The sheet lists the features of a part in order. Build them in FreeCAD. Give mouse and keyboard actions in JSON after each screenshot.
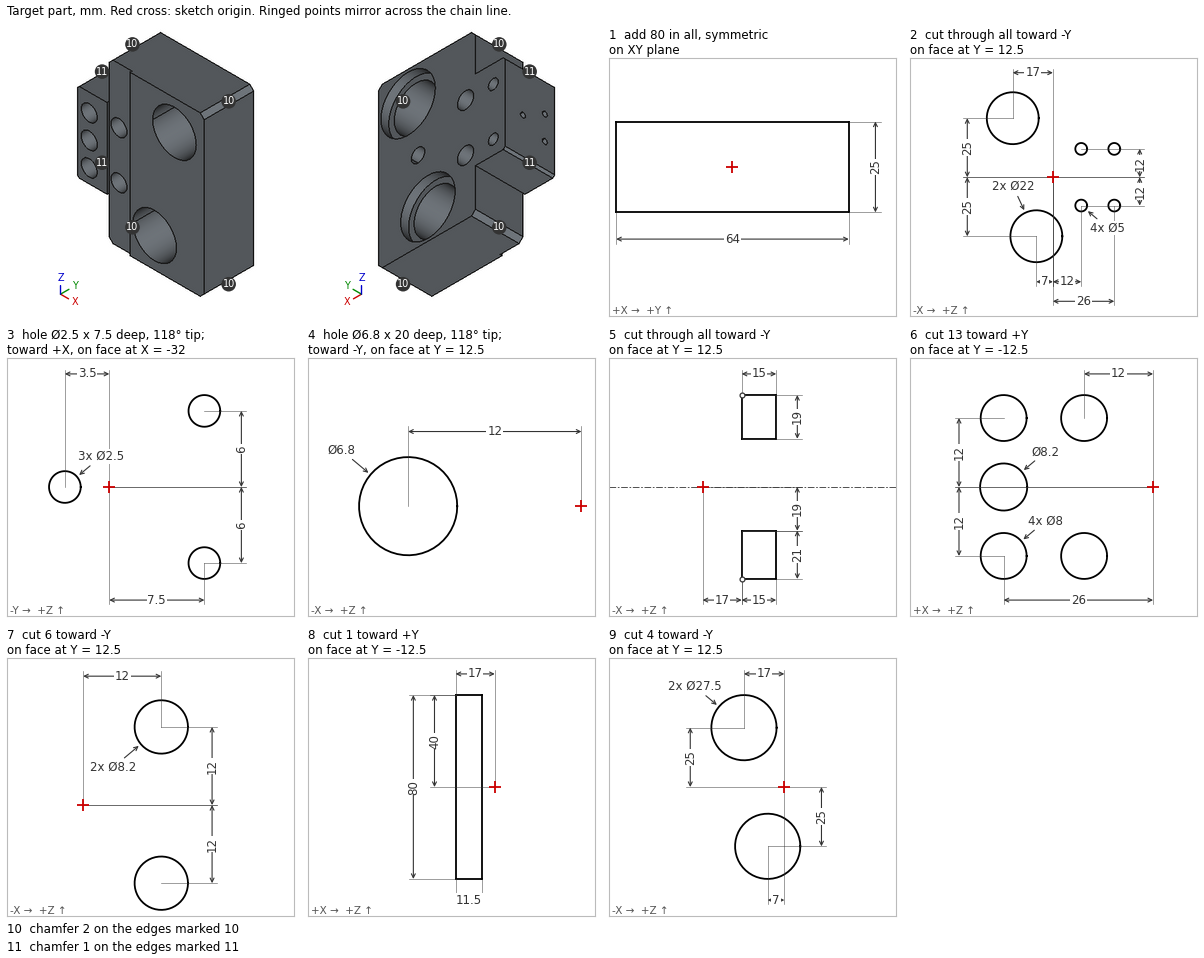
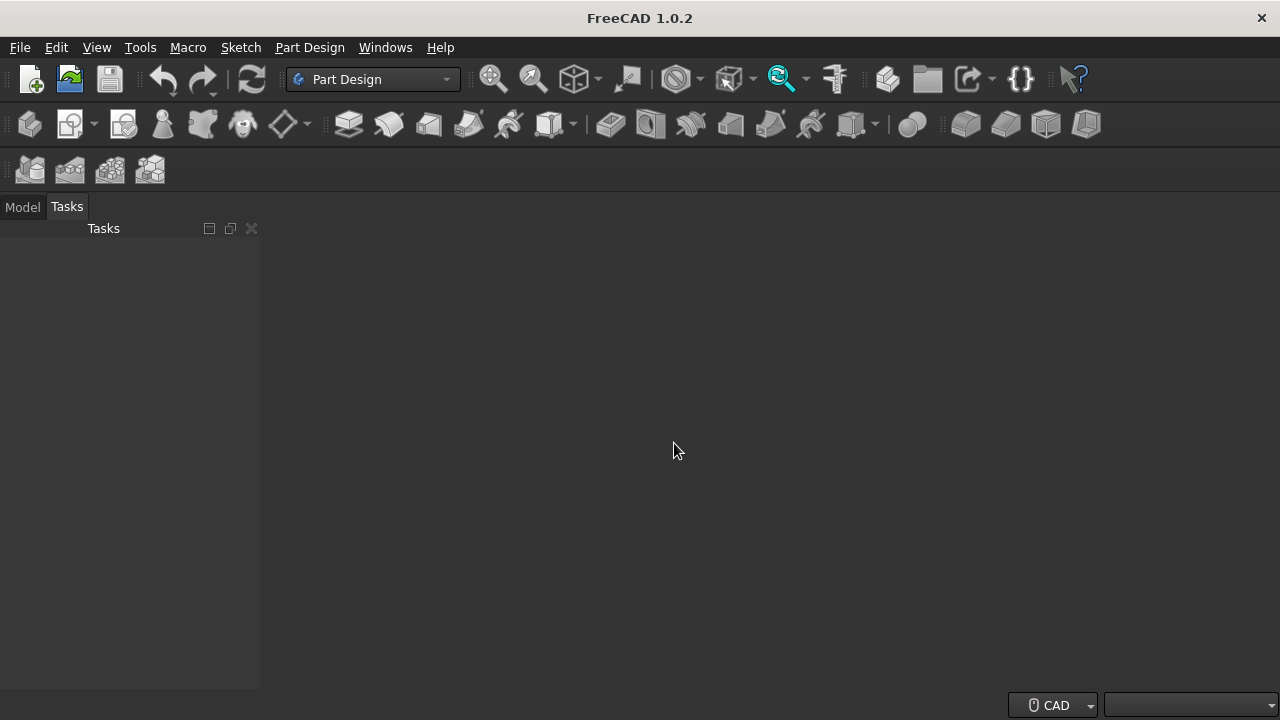
{"action": "left_click", "coordinate": [30, 80]}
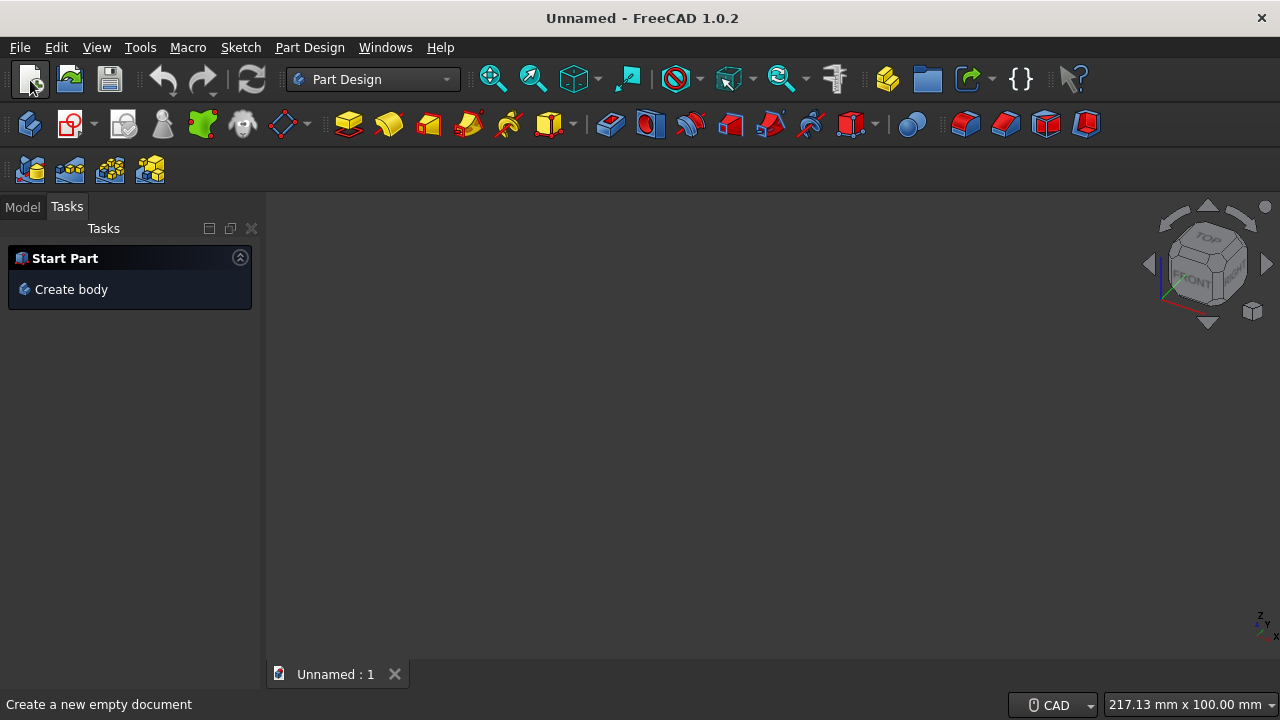
{"action": "left_click", "coordinate": [70, 124]}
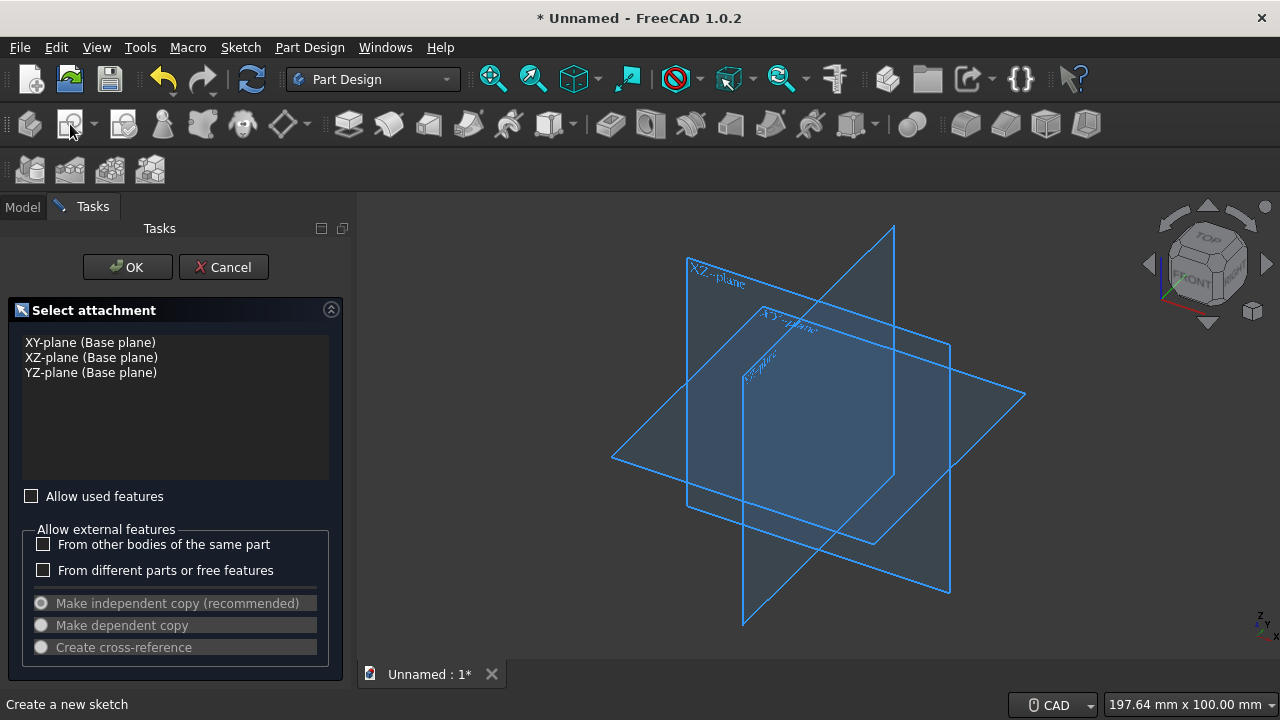
{"action": "left_click", "coordinate": [82, 342]}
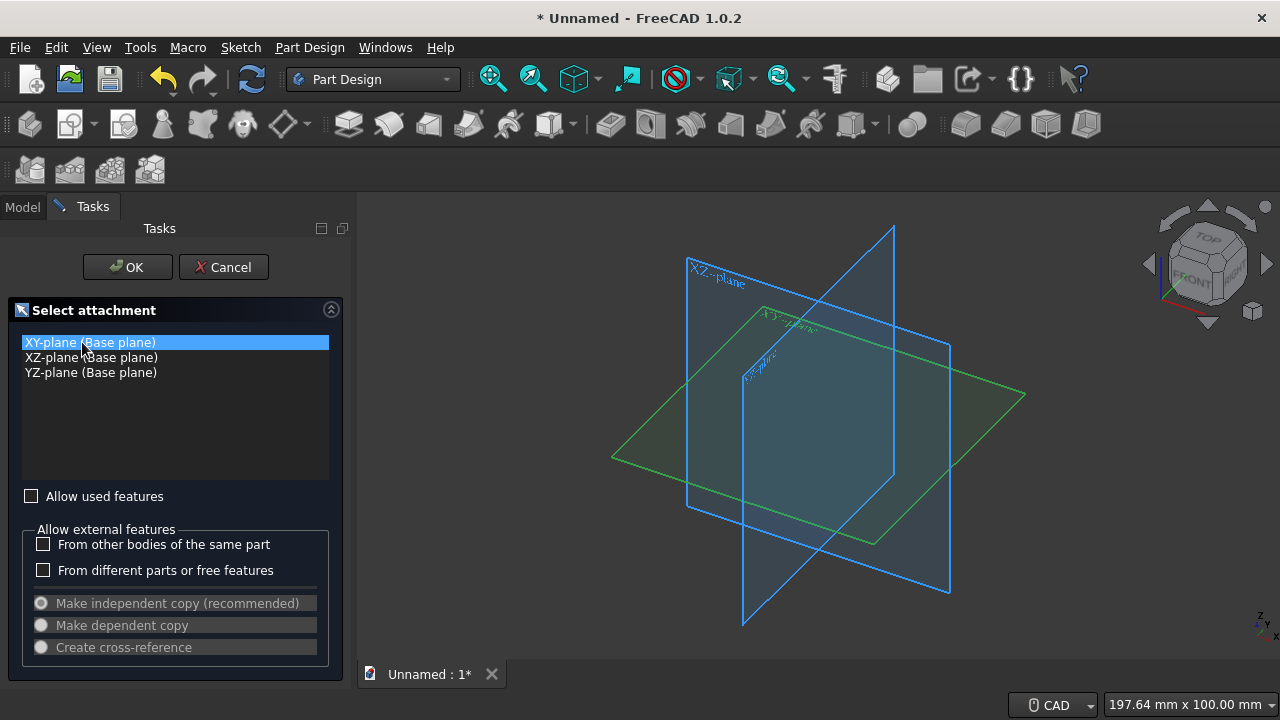
{"action": "left_click", "coordinate": [128, 267]}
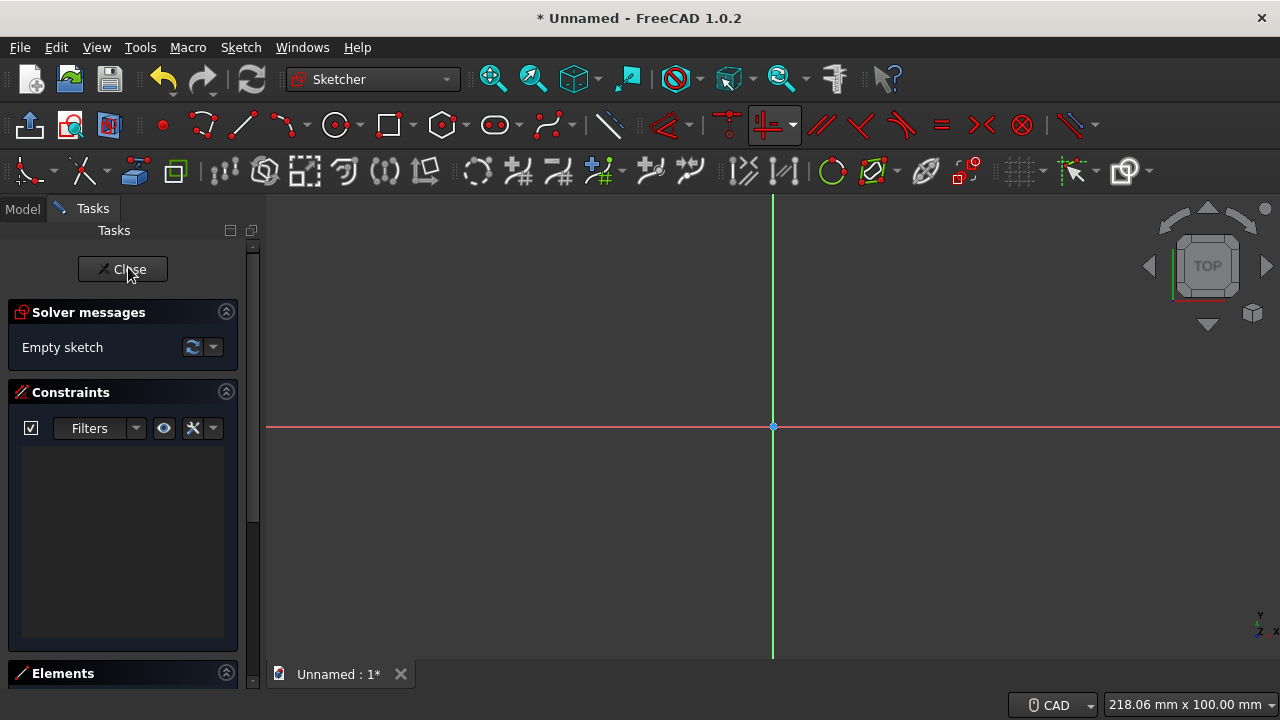
{"action": "scroll", "coordinate": [856, 426], "scroll_direction": "up", "scroll_amount": 3}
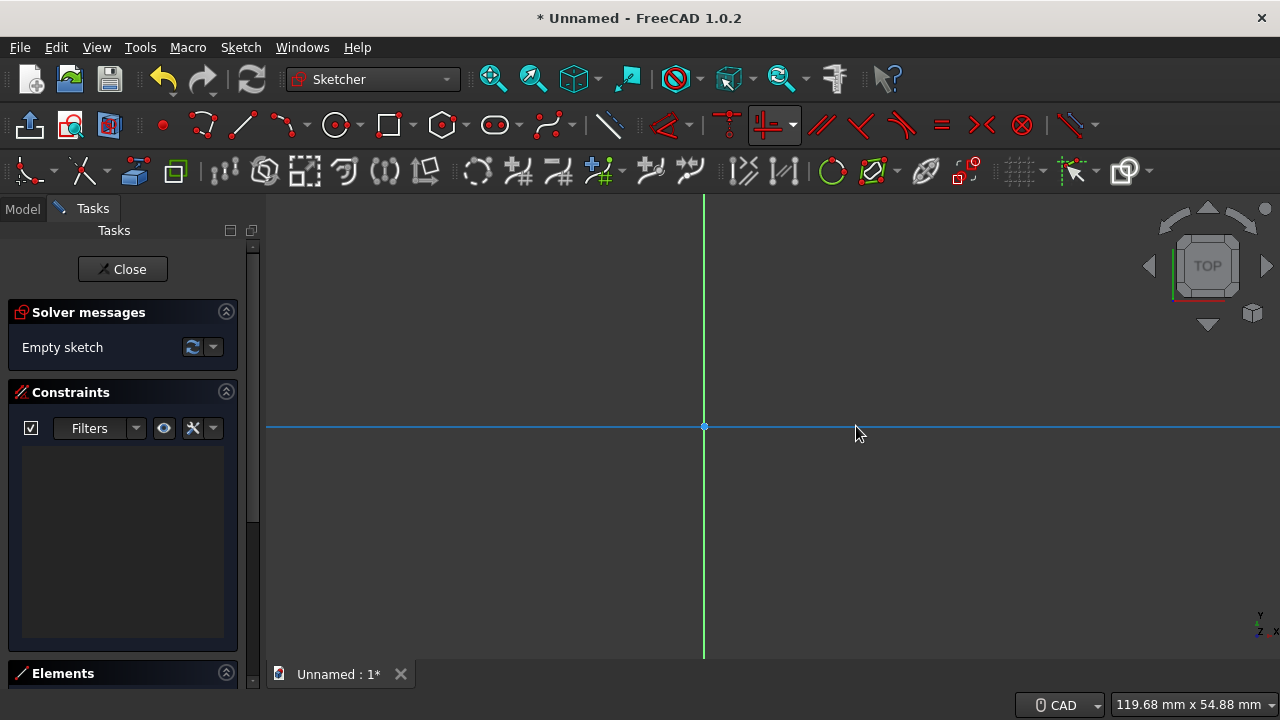
{"action": "left_click", "coordinate": [416, 126]}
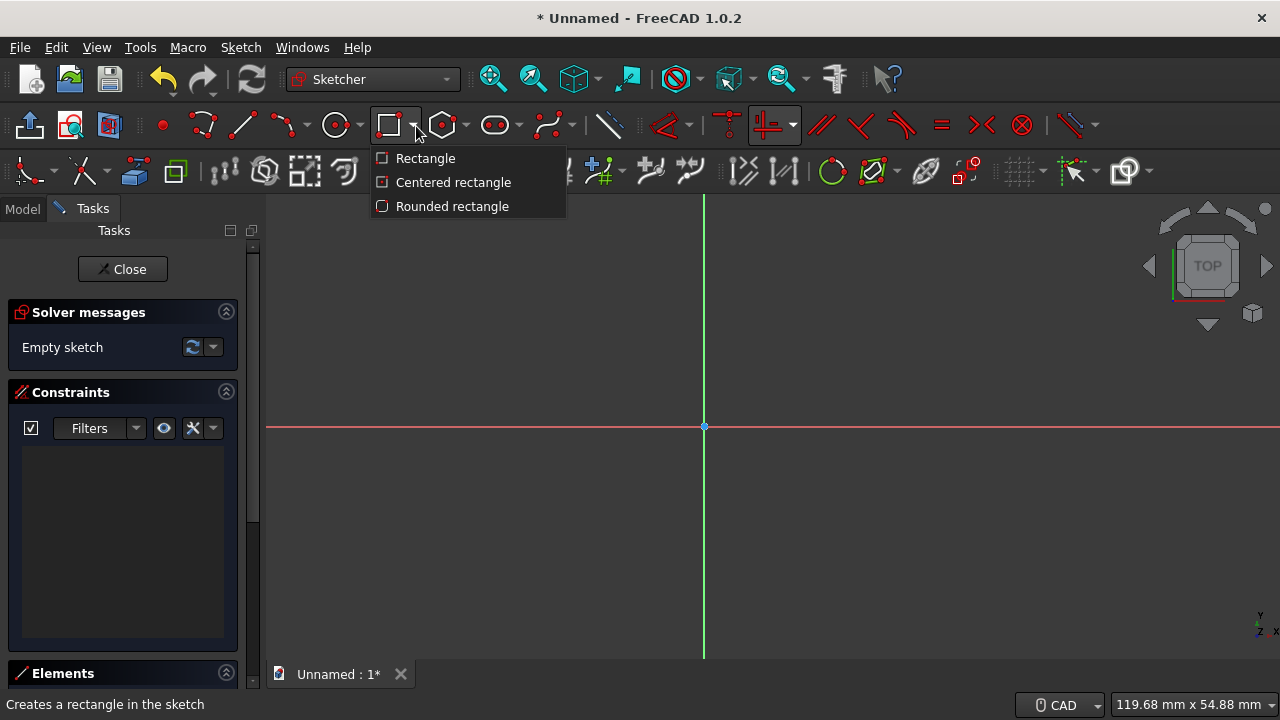
{"action": "left_click", "coordinate": [468, 182]}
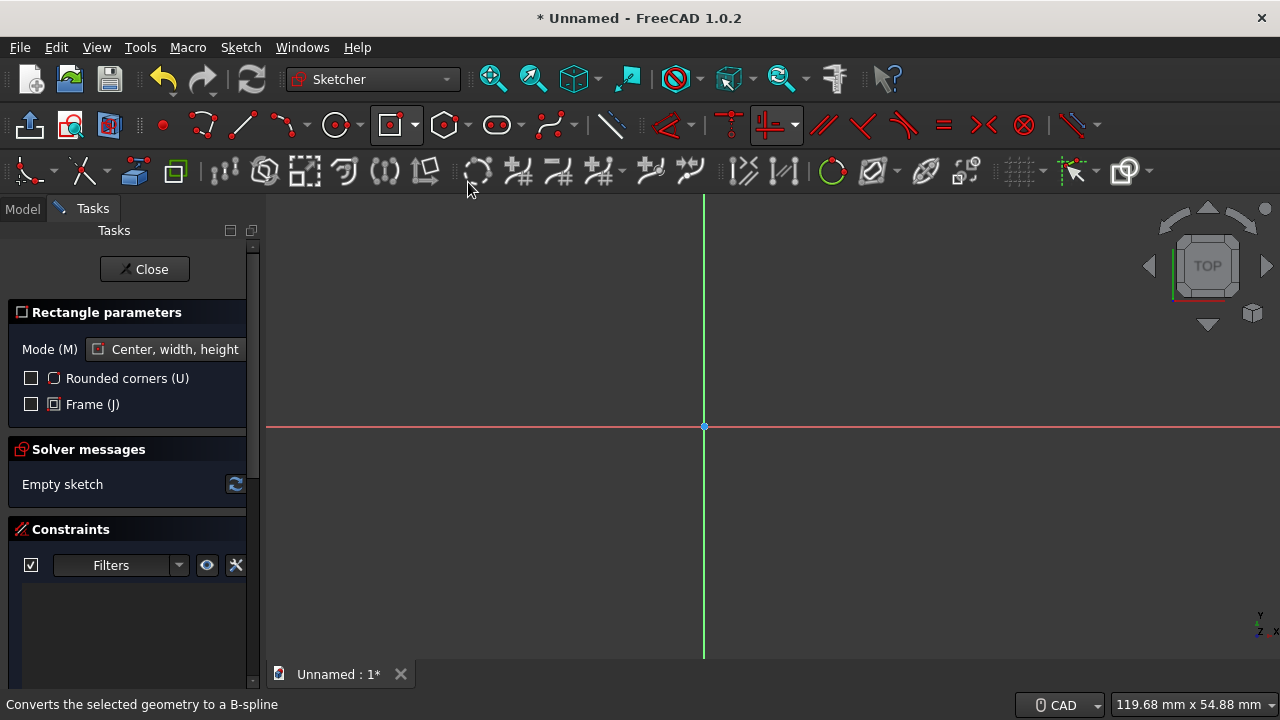
{"action": "left_click", "coordinate": [704, 426]}
{"action": "left_click", "coordinate": [975, 321]}
{"action": "key", "text": "Escape"}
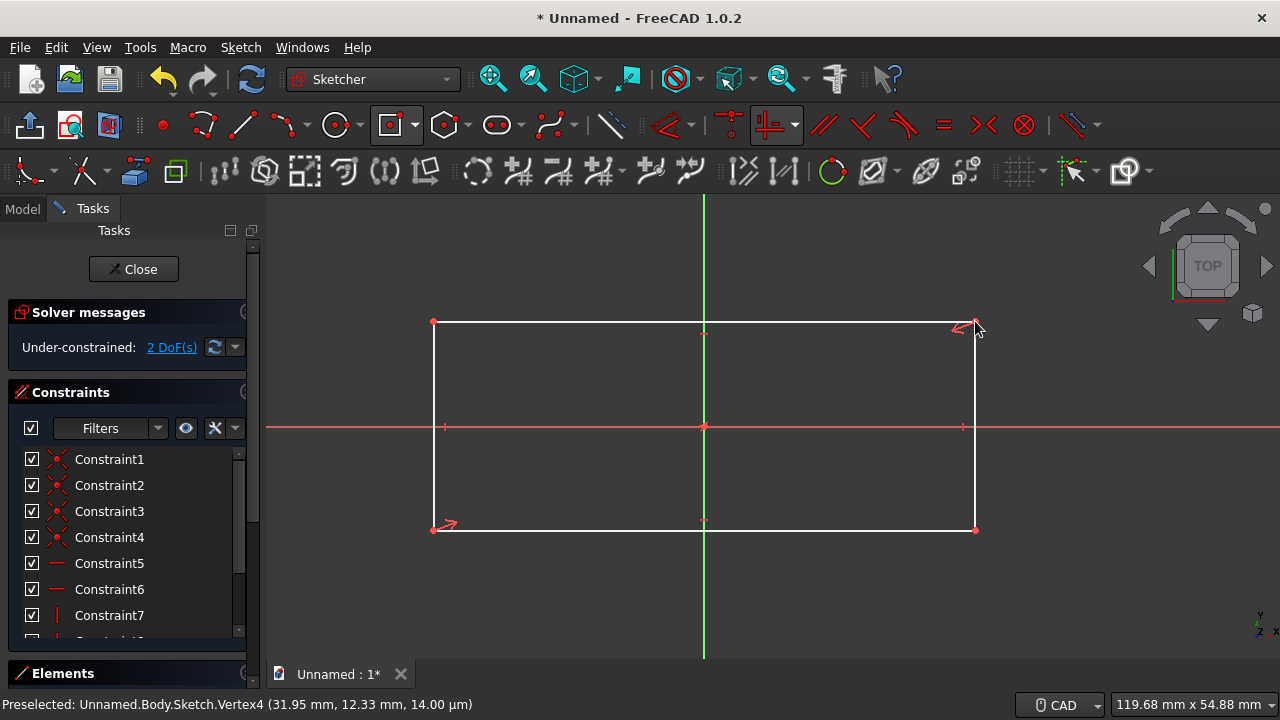
{"action": "left_click", "coordinate": [666, 126]}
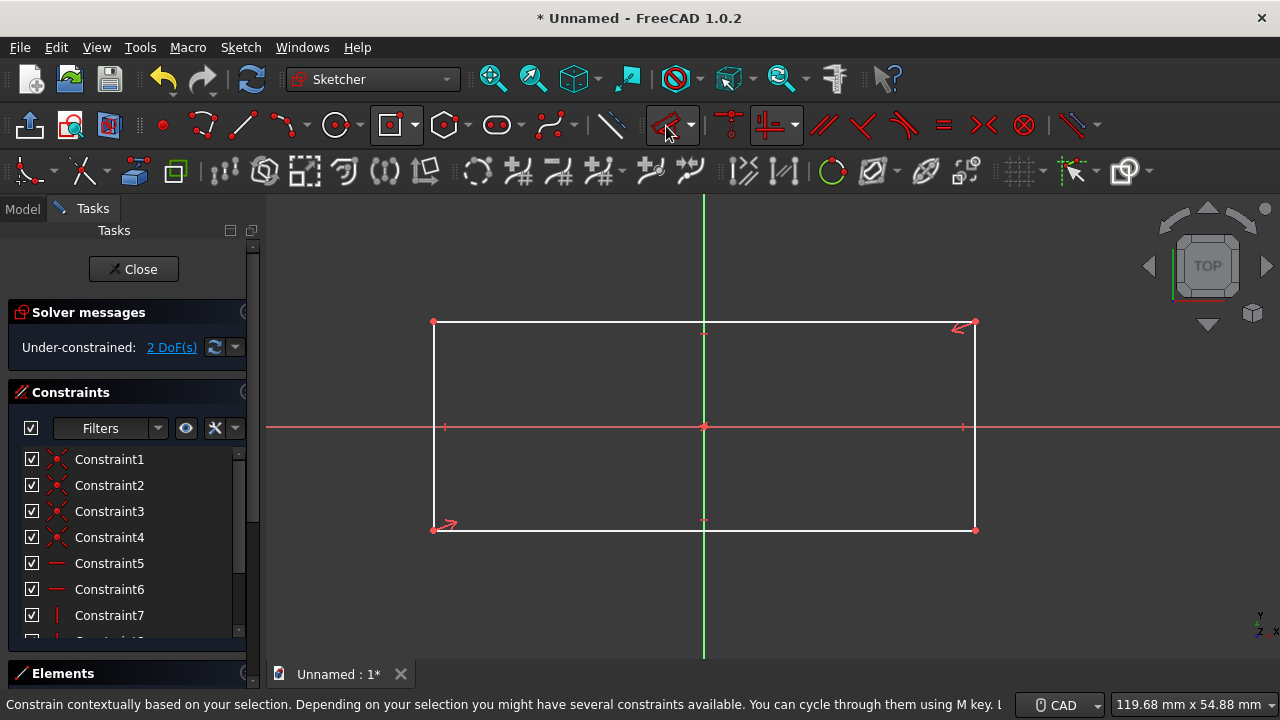
{"action": "left_click", "coordinate": [596, 531]}
{"action": "left_click", "coordinate": [580, 565]}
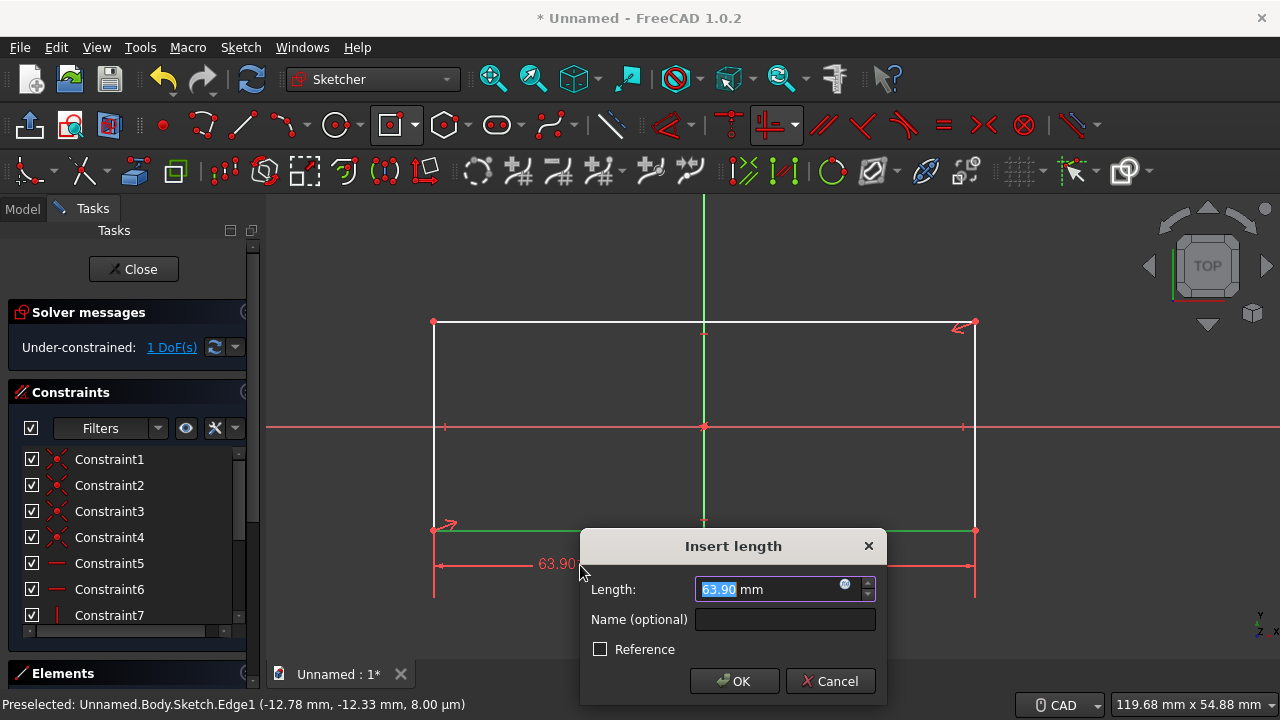
{"action": "type", "text": "64"}
{"action": "key", "text": "Return"}